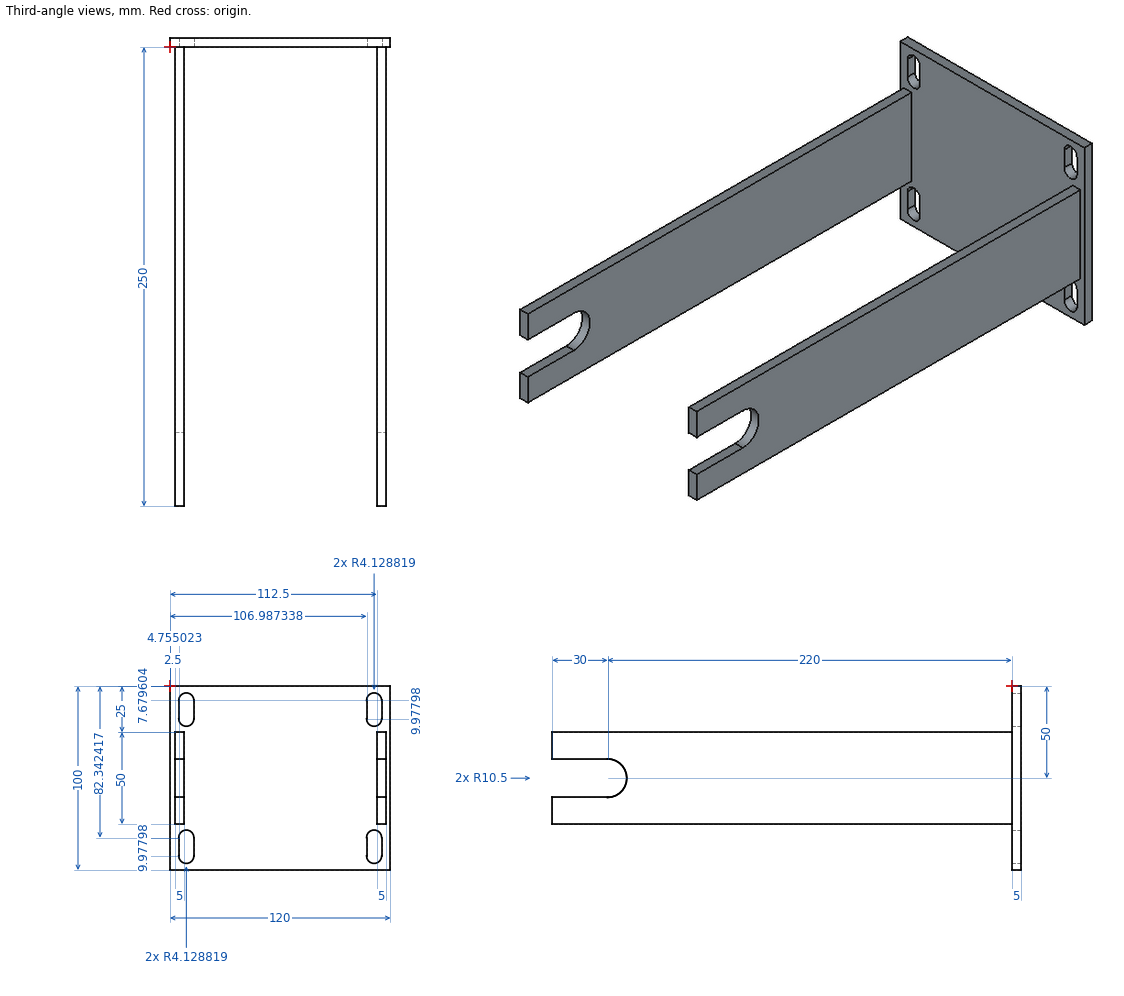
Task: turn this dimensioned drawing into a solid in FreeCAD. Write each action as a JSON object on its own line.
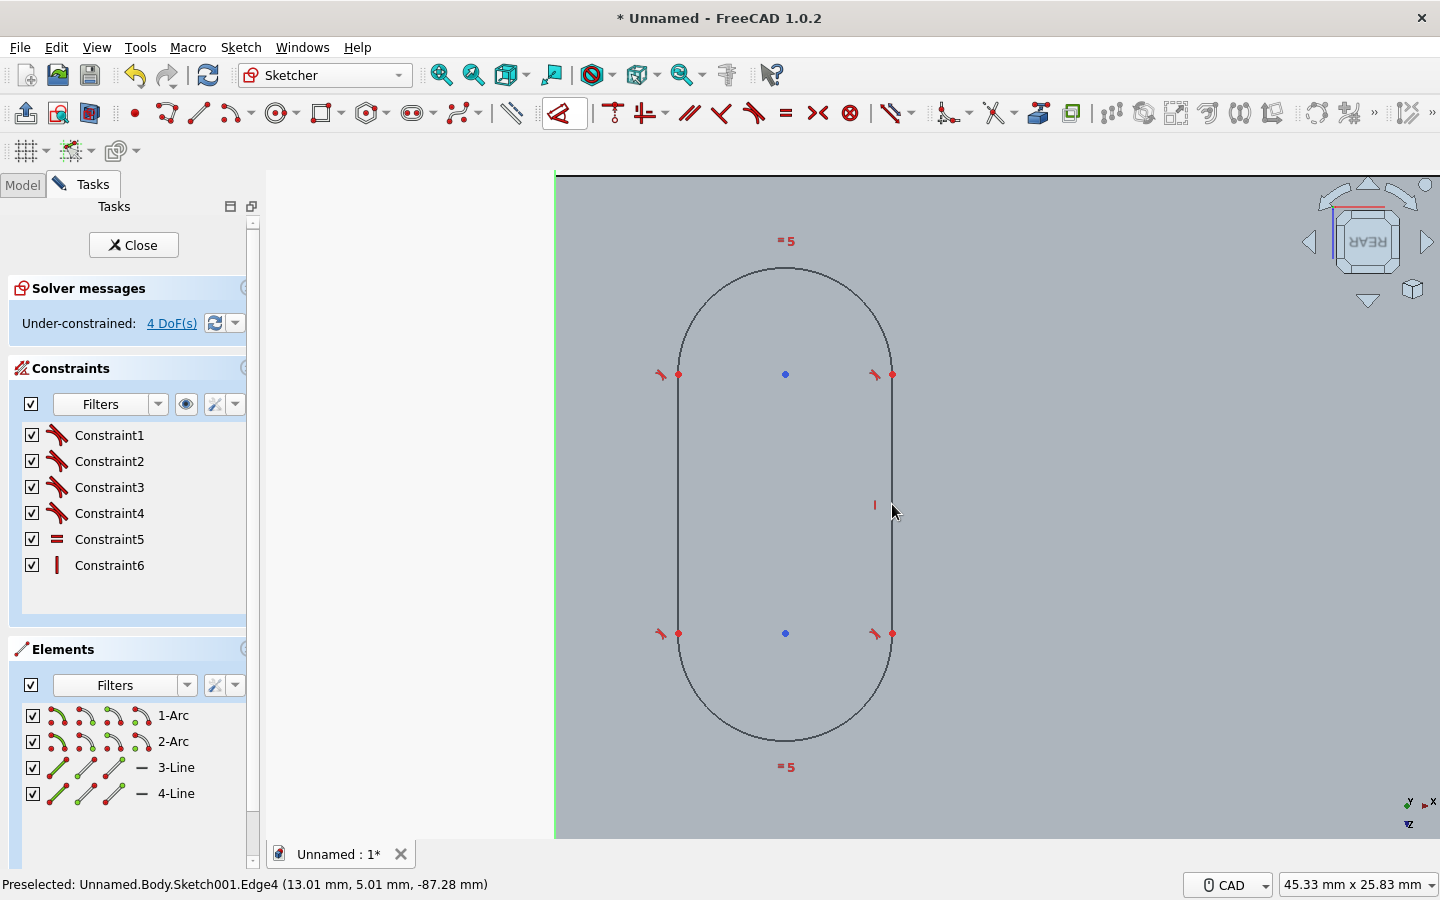
{"action": "left_click", "coordinate": [722, 721]}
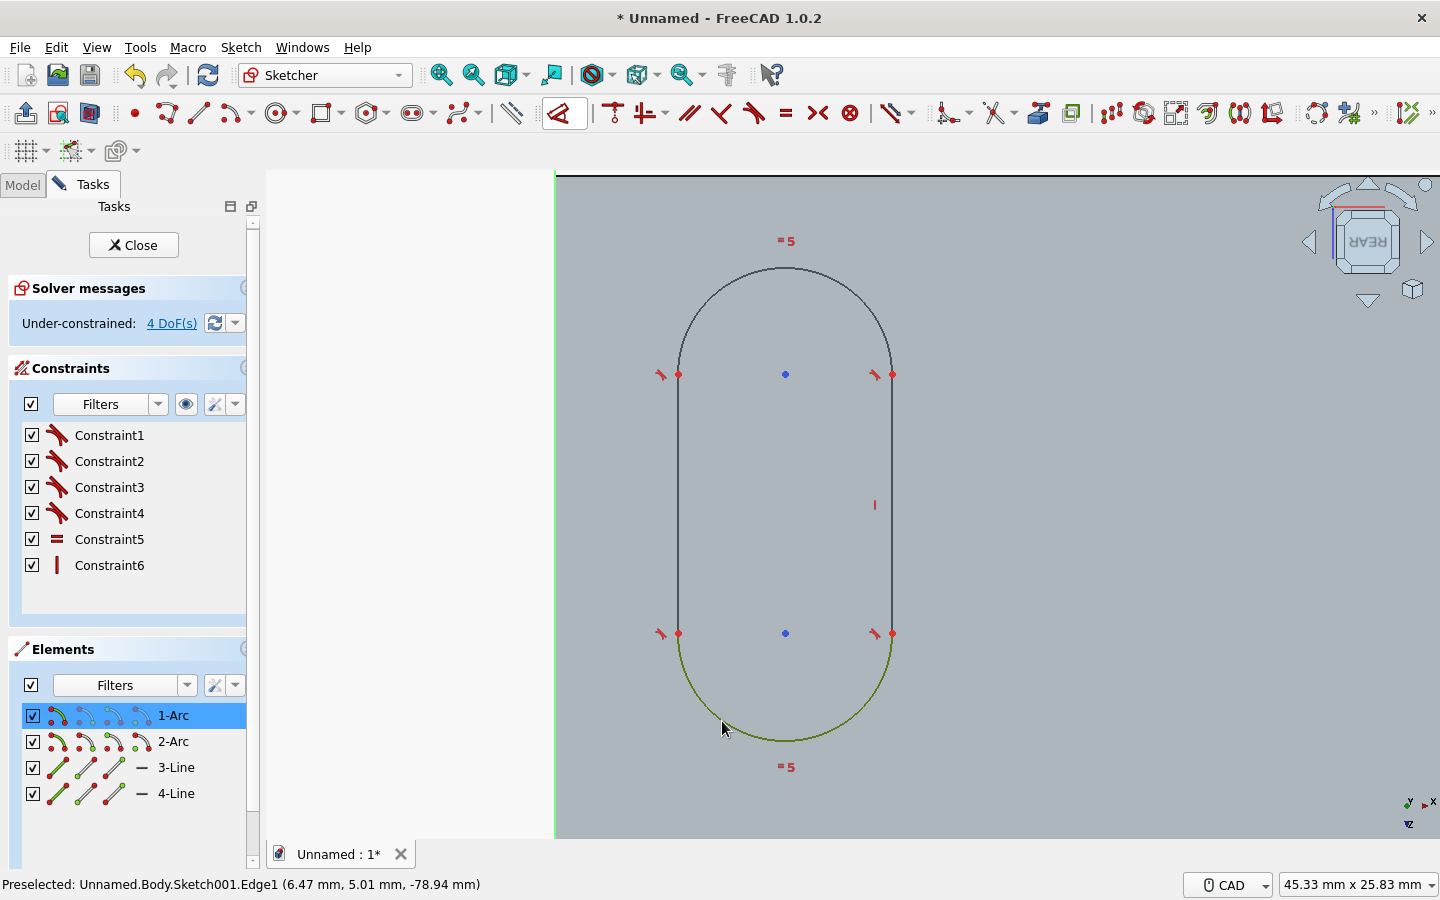
{"action": "key", "text": "k r"}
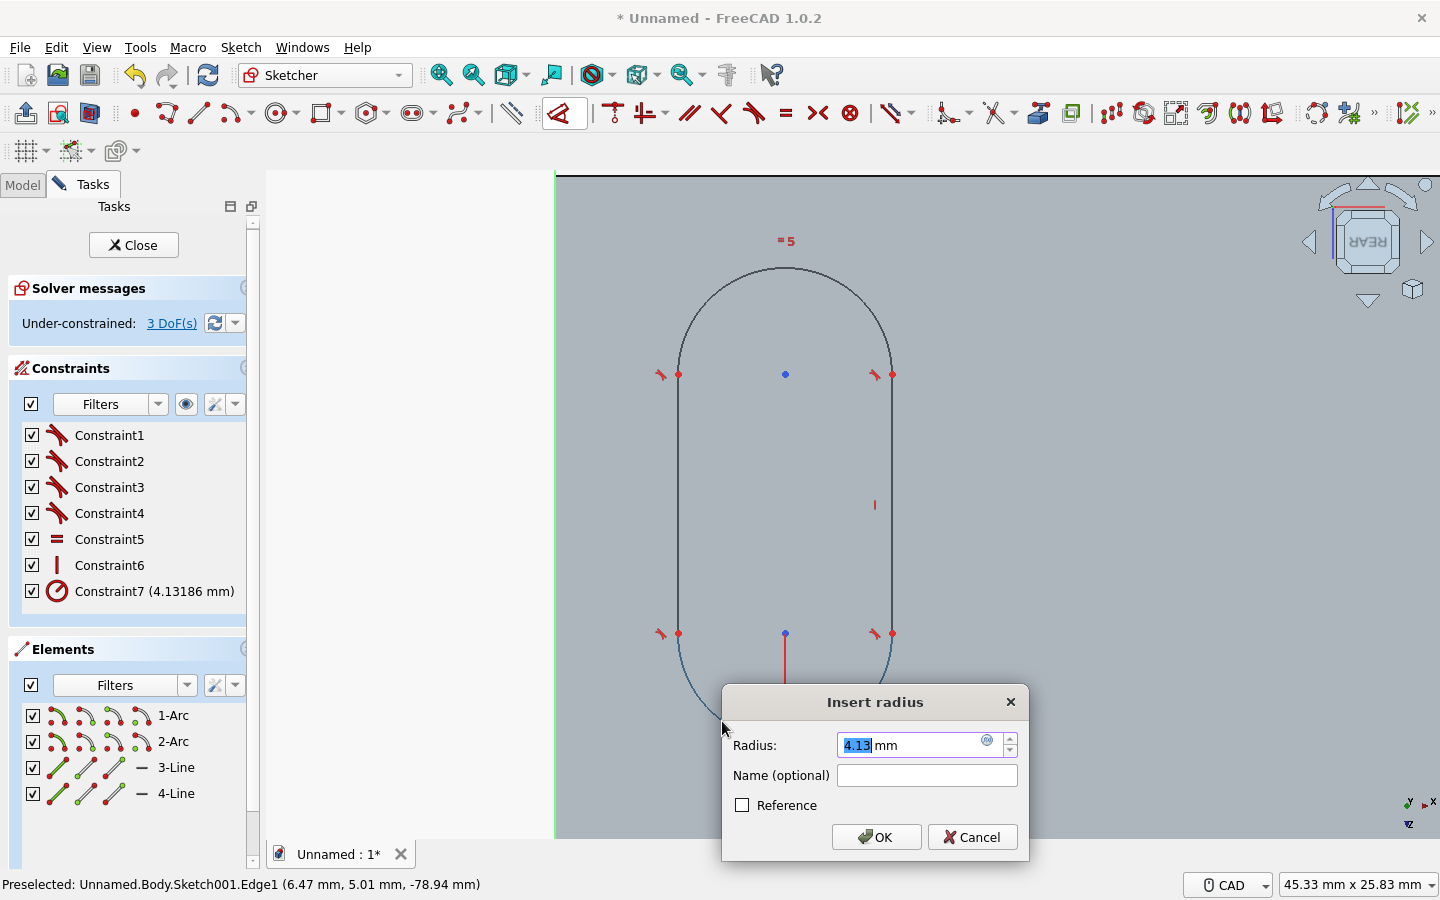
{"action": "type", "text": "4.128819"}
{"action": "key", "text": "Return"}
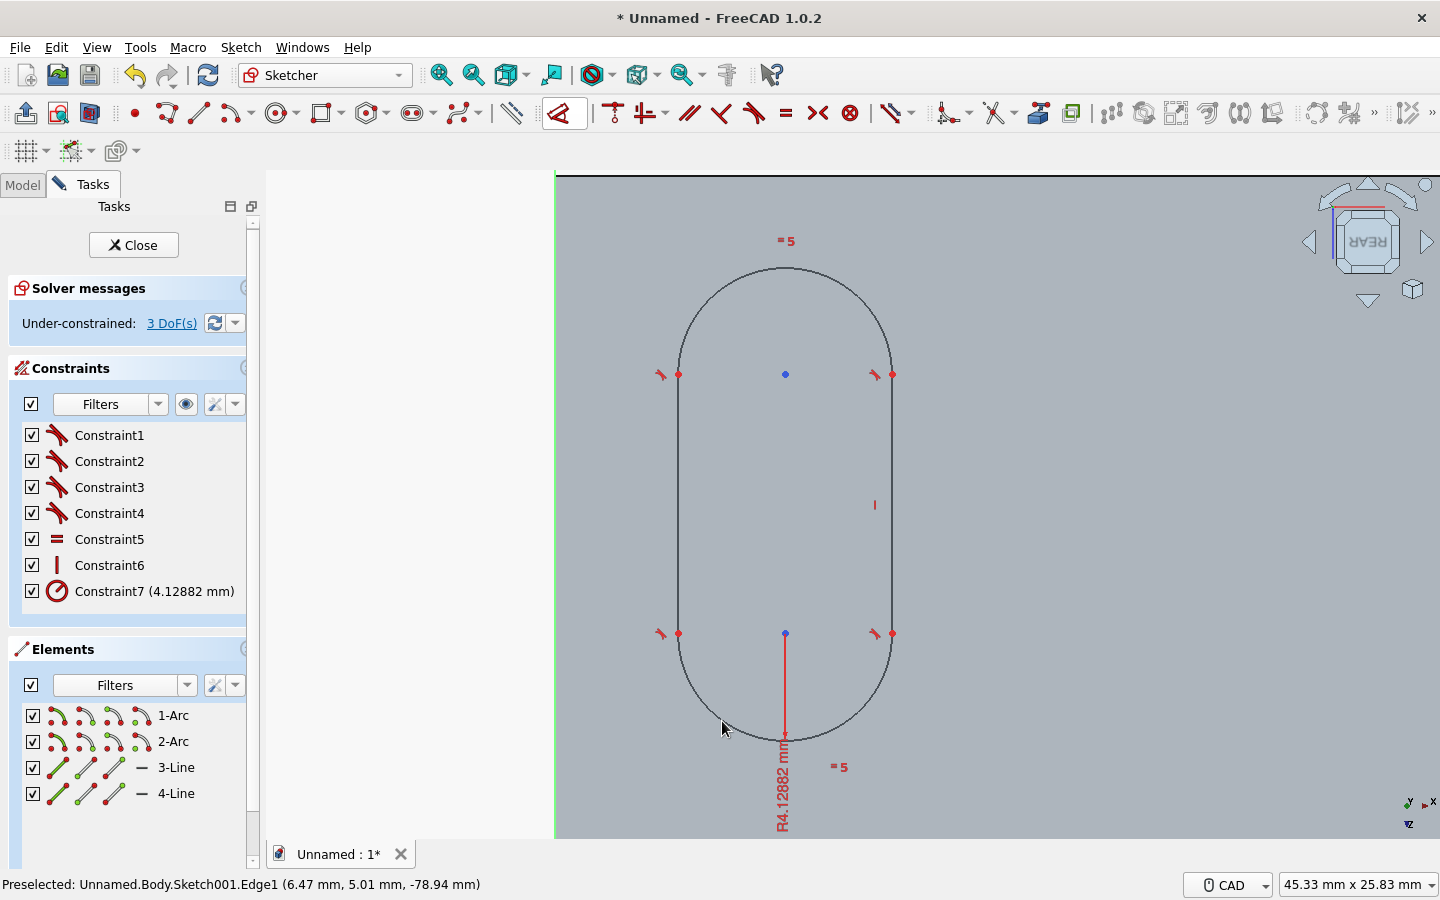
{"action": "left_click", "coordinate": [678, 556]}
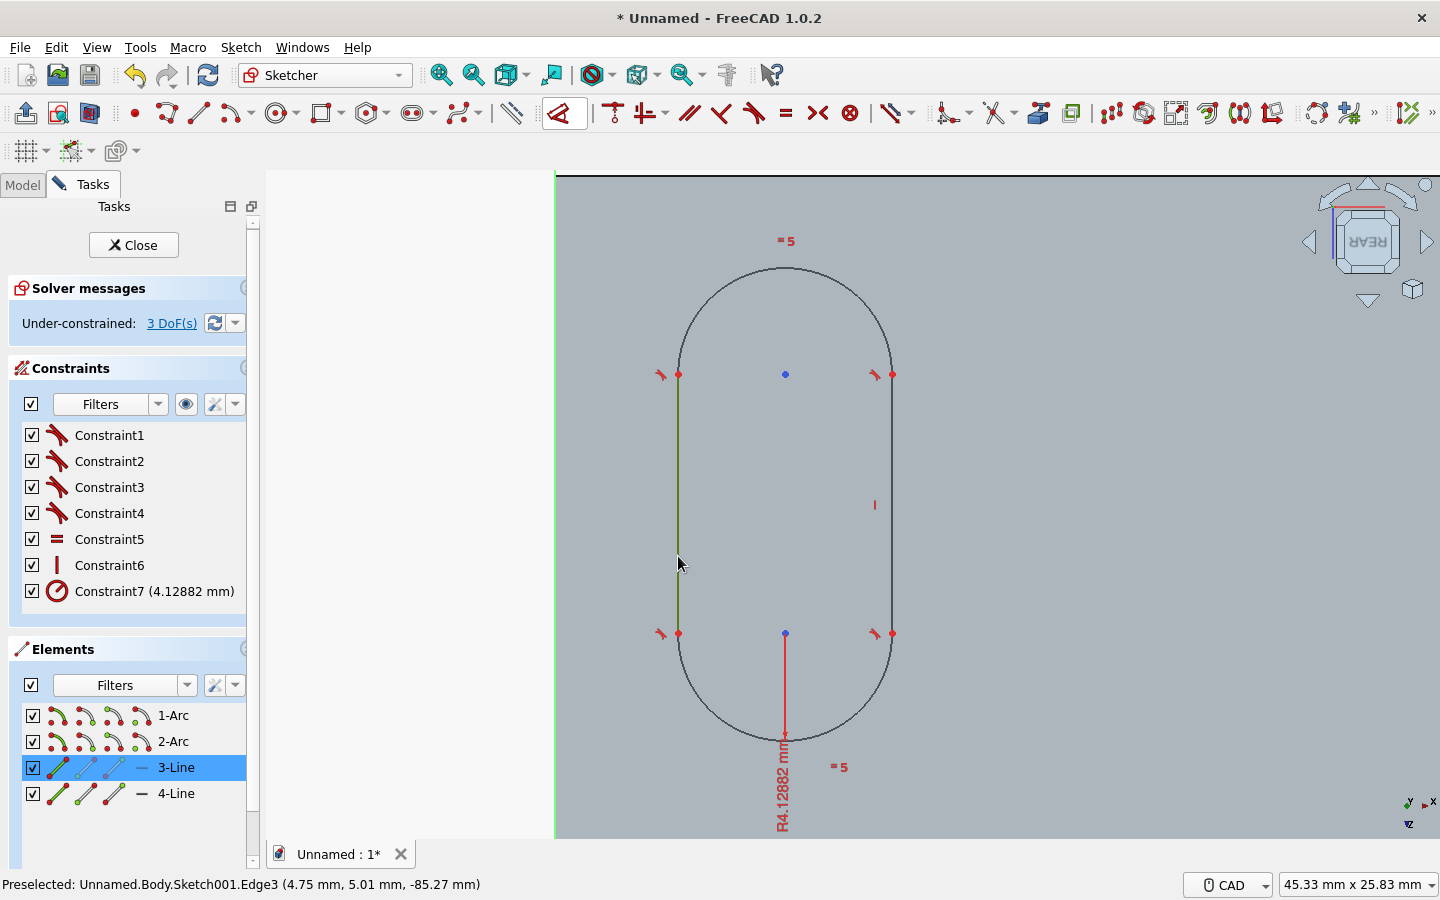
{"action": "left_click", "coordinate": [582, 114]}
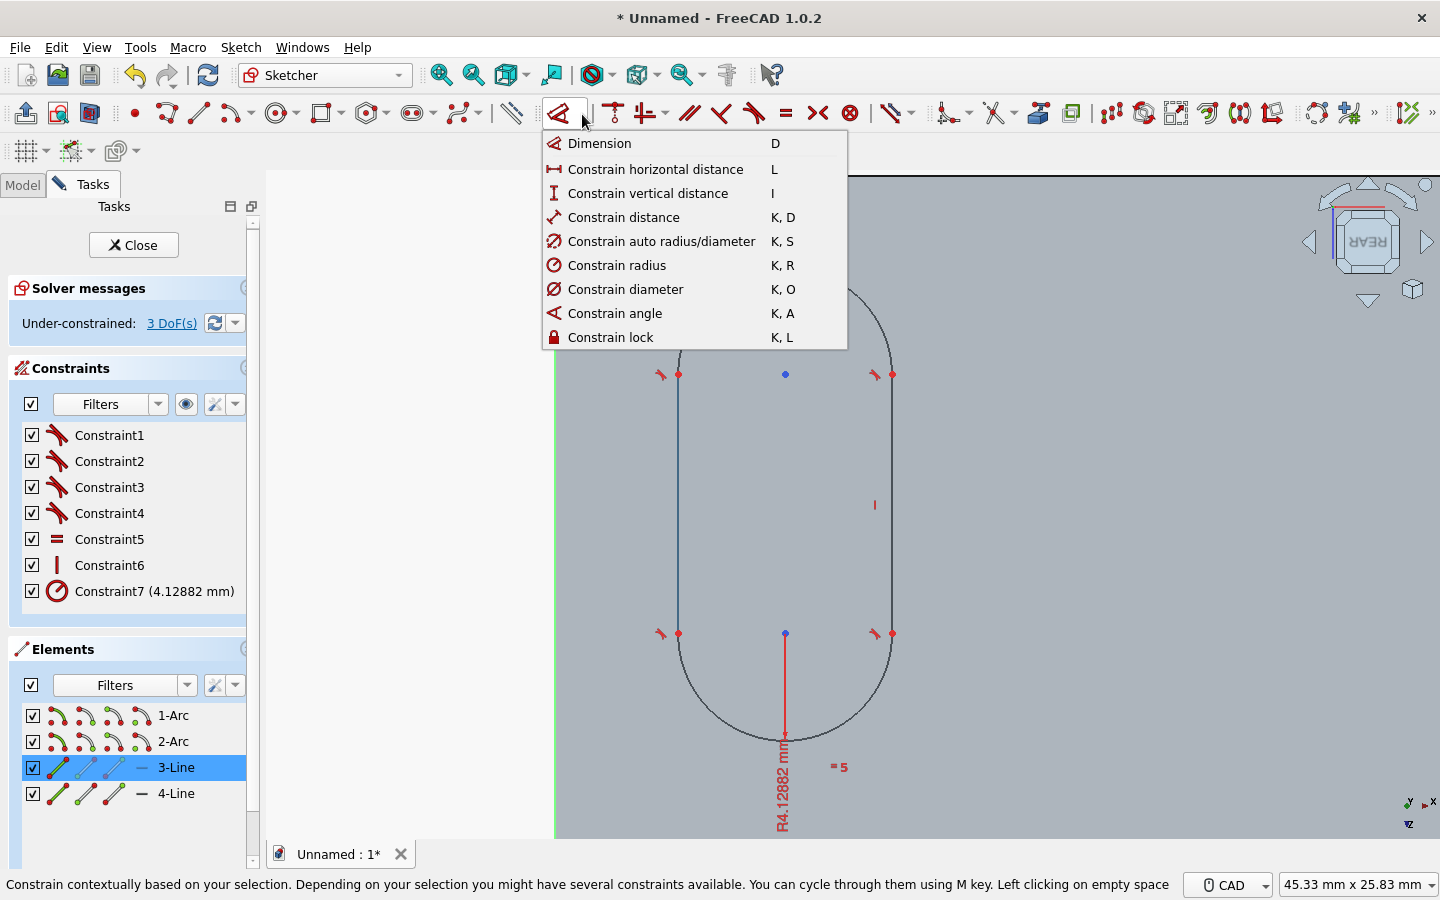
{"action": "left_click", "coordinate": [695, 193]}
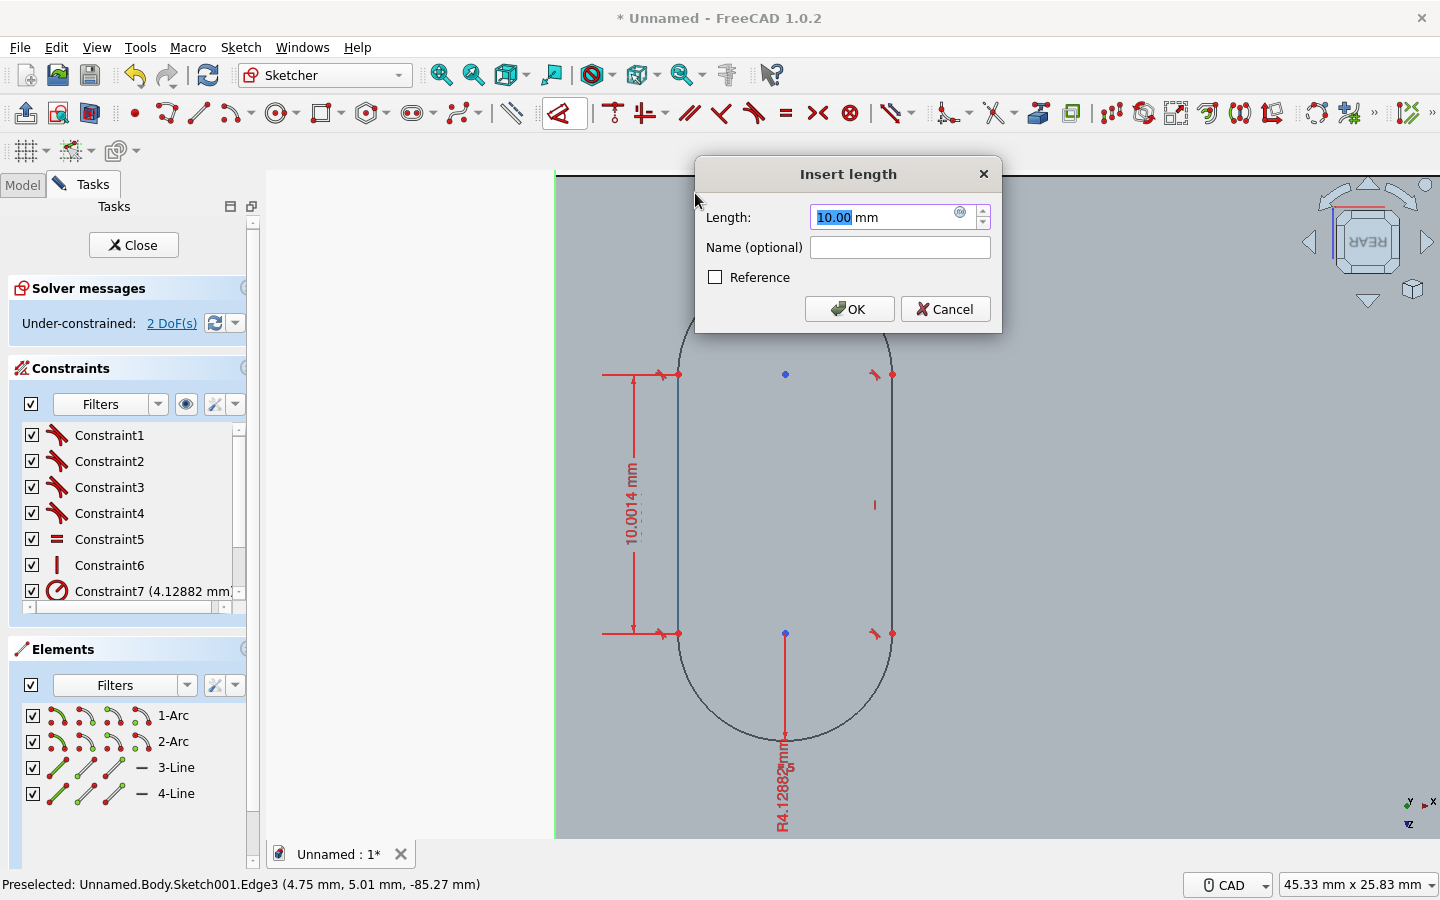
{"action": "type", "text": "9.97798"}
{"action": "key", "text": "Return"}